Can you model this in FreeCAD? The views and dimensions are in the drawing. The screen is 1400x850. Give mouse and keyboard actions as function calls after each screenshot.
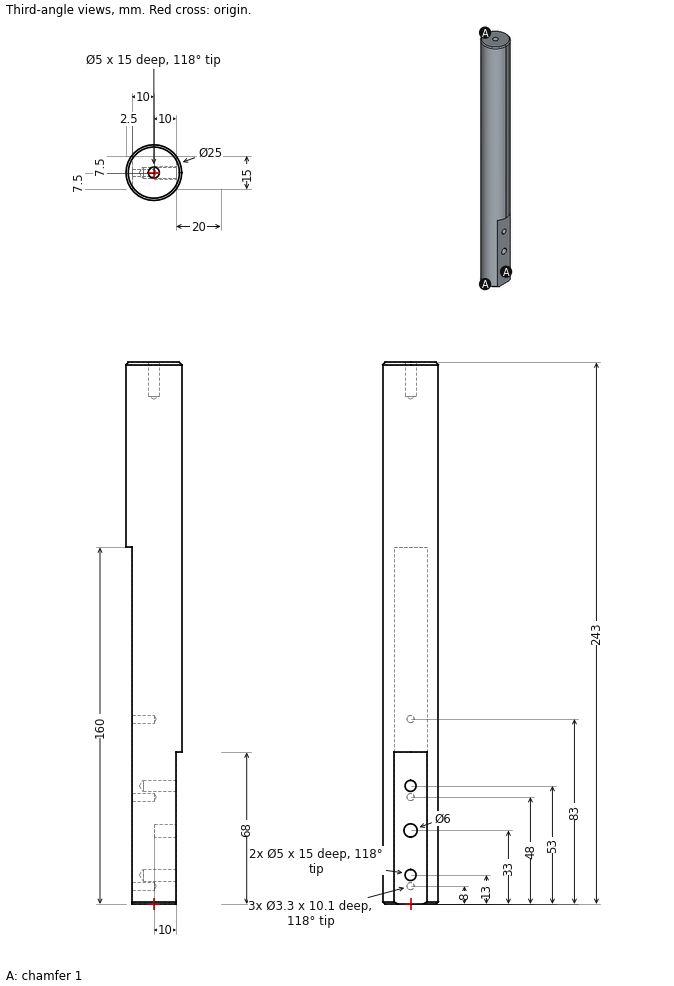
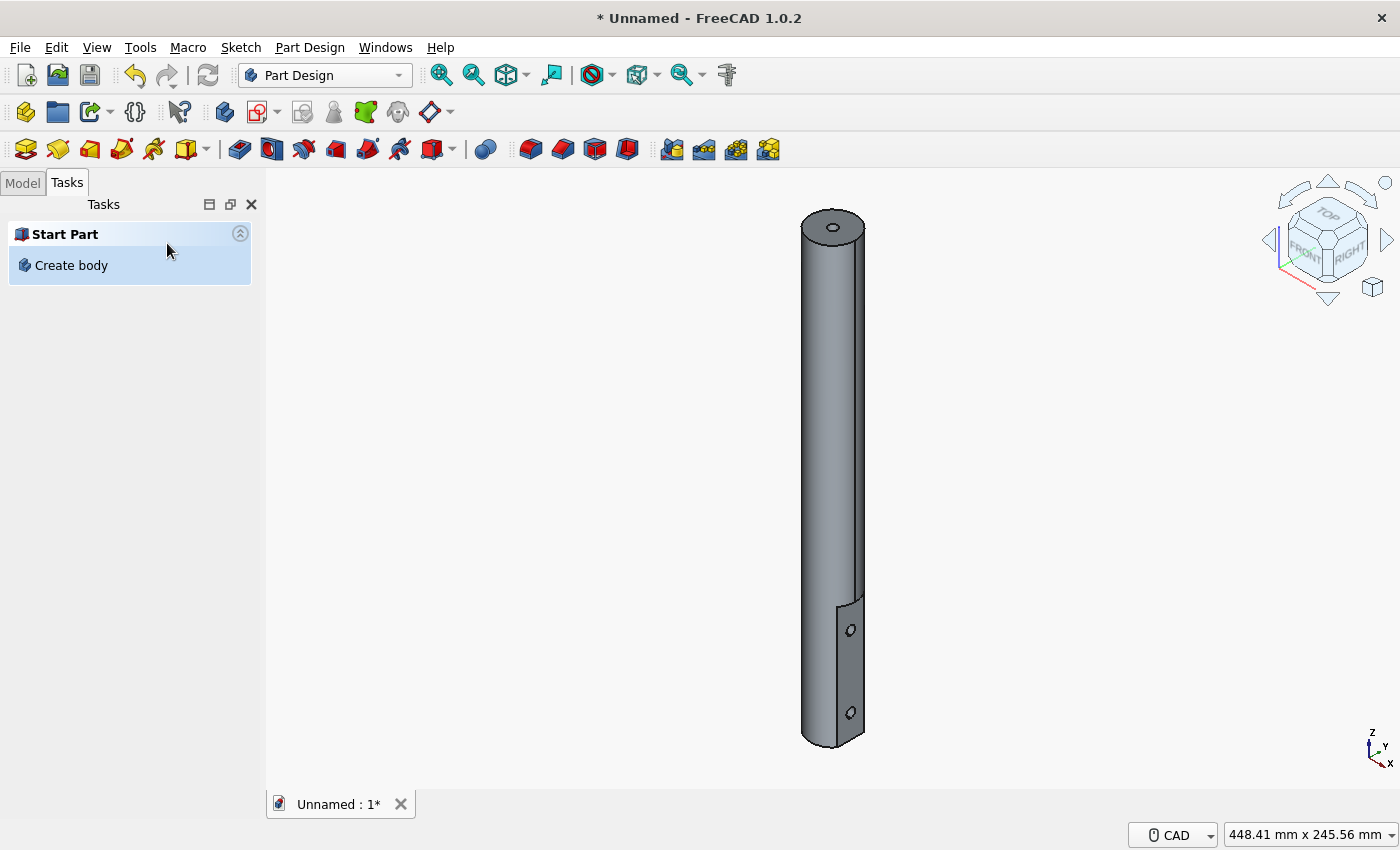
click(851, 668)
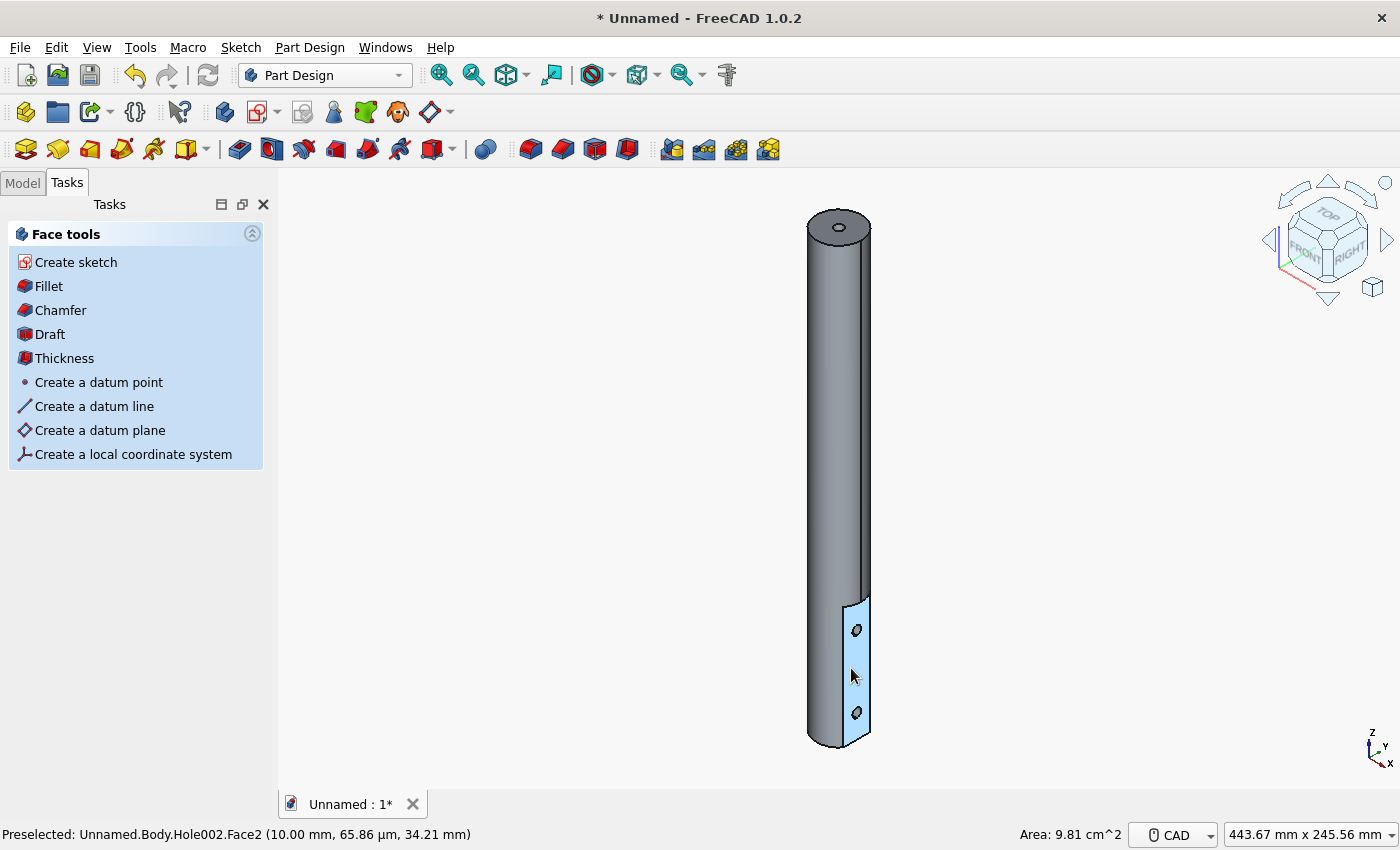
click(258, 112)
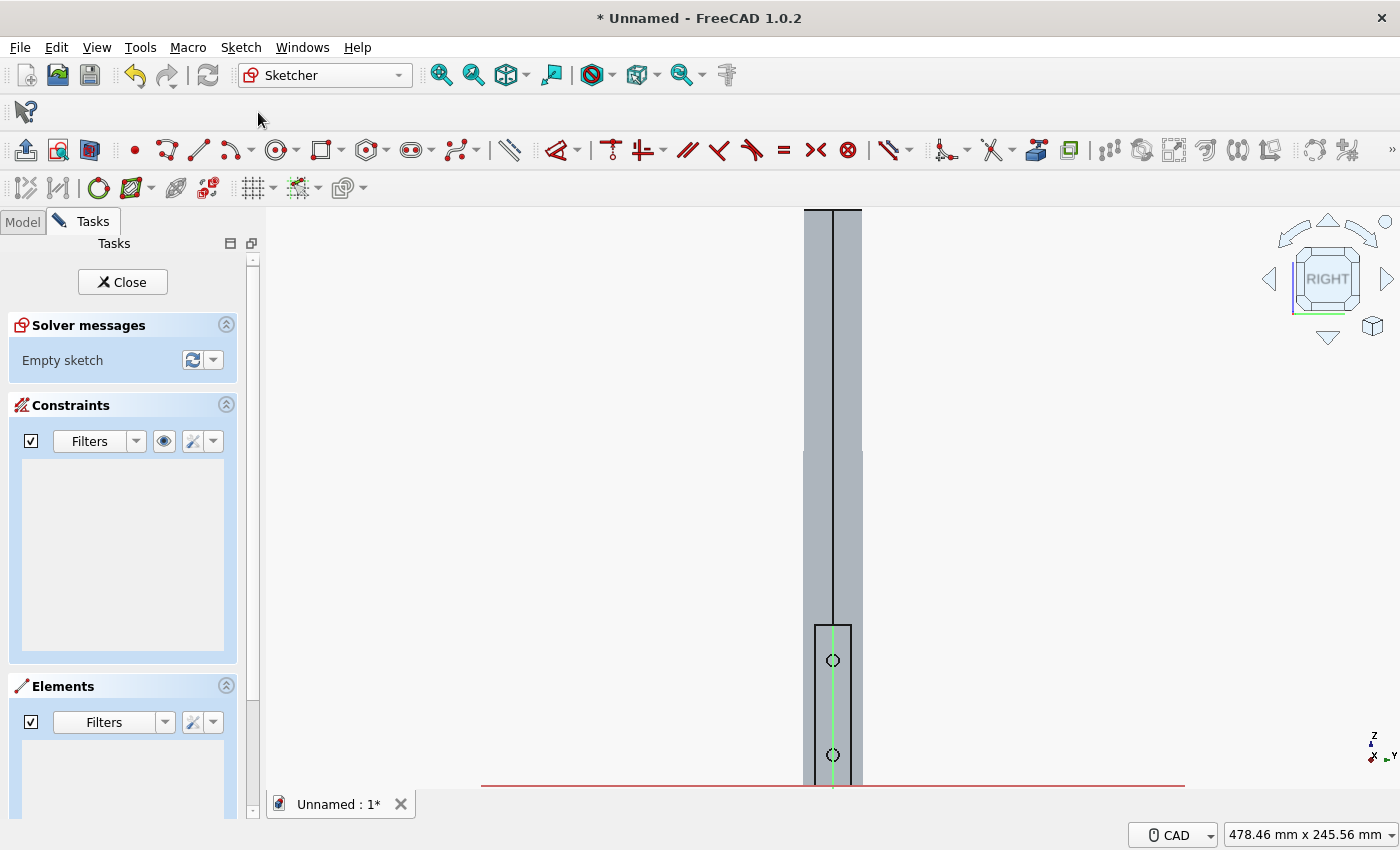
key(q)
key(s)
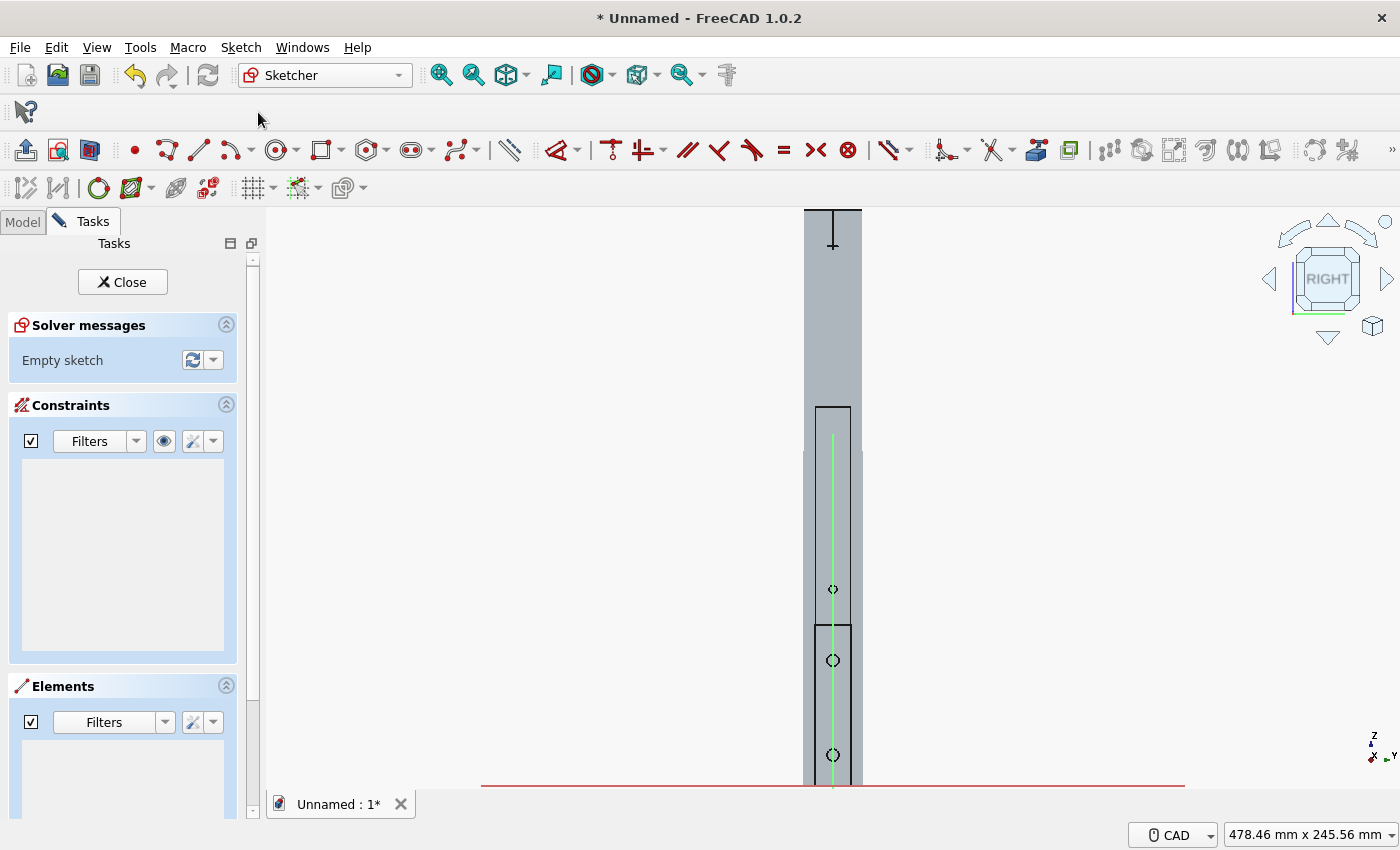
scroll(837, 719, up, 15)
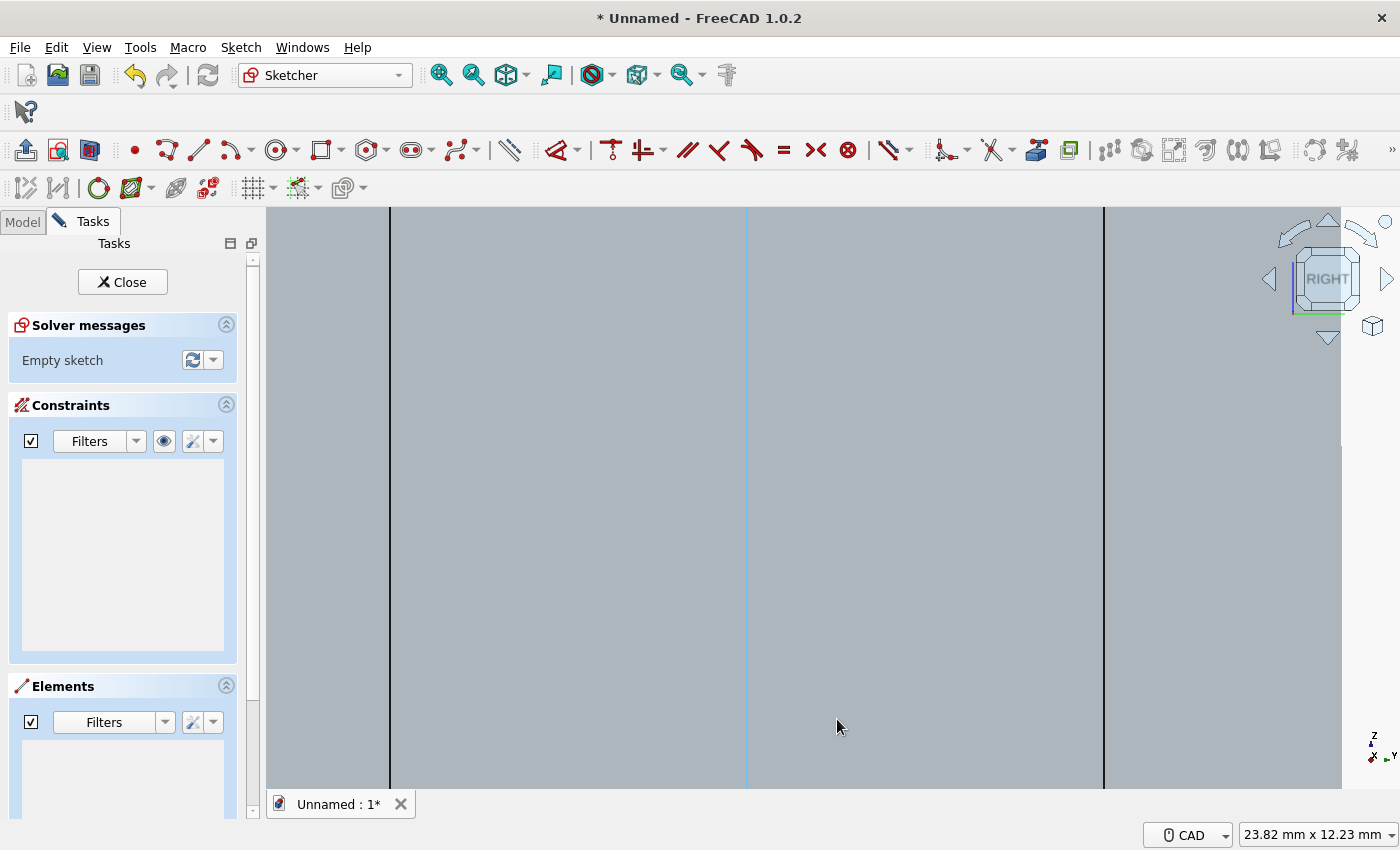
key(g)
key(c)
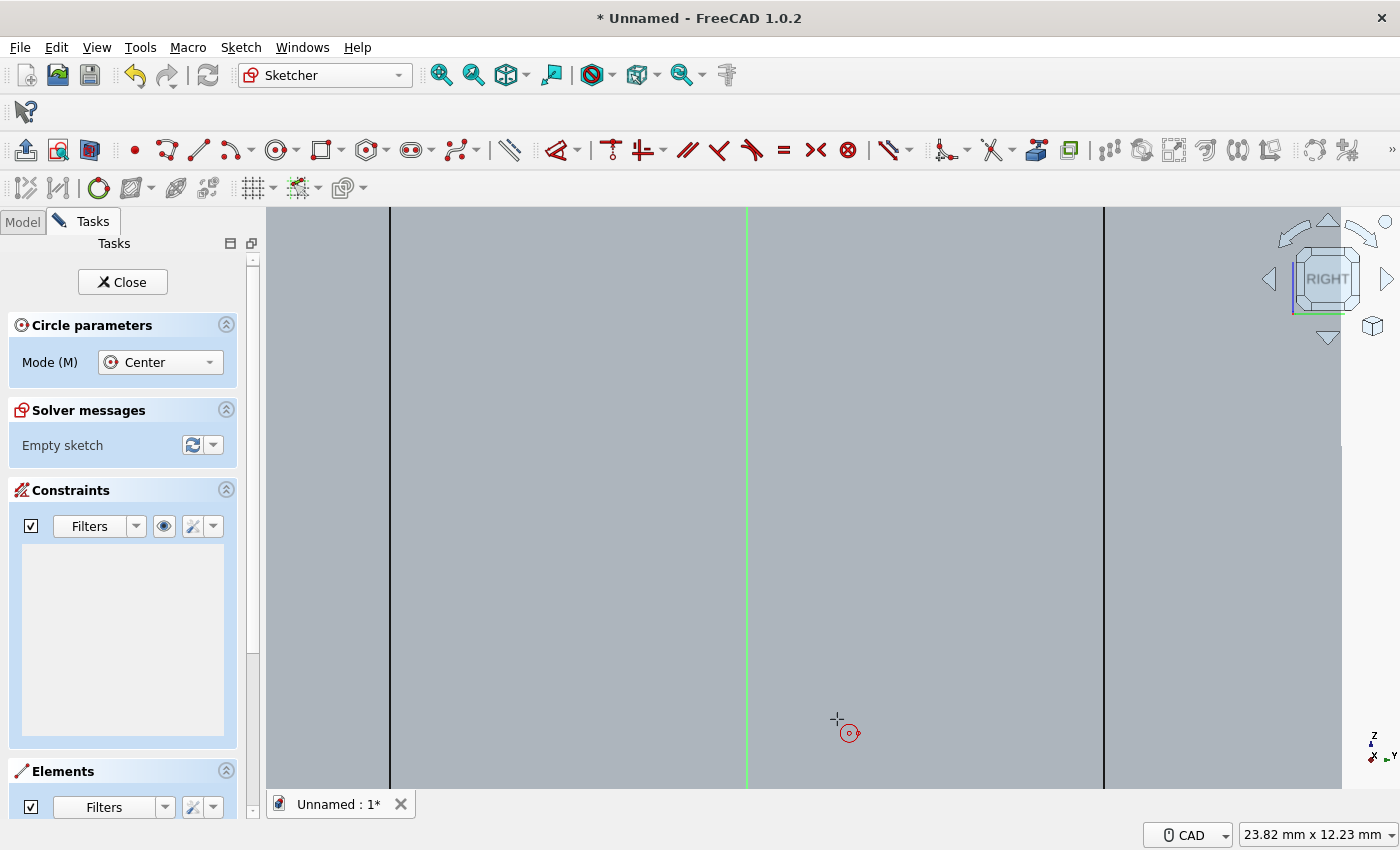
click(747, 476)
click(848, 375)
key(Escape)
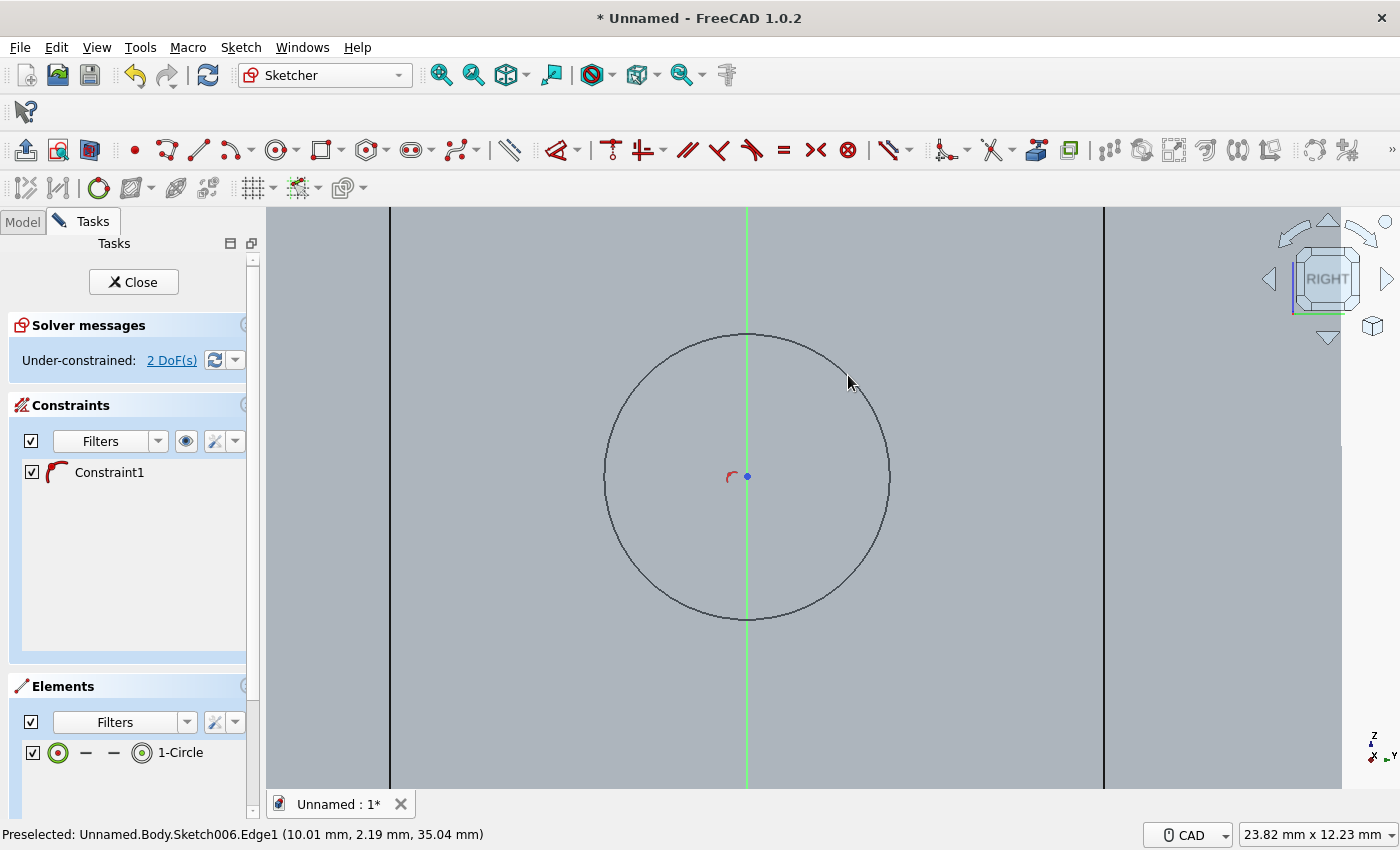
key(d)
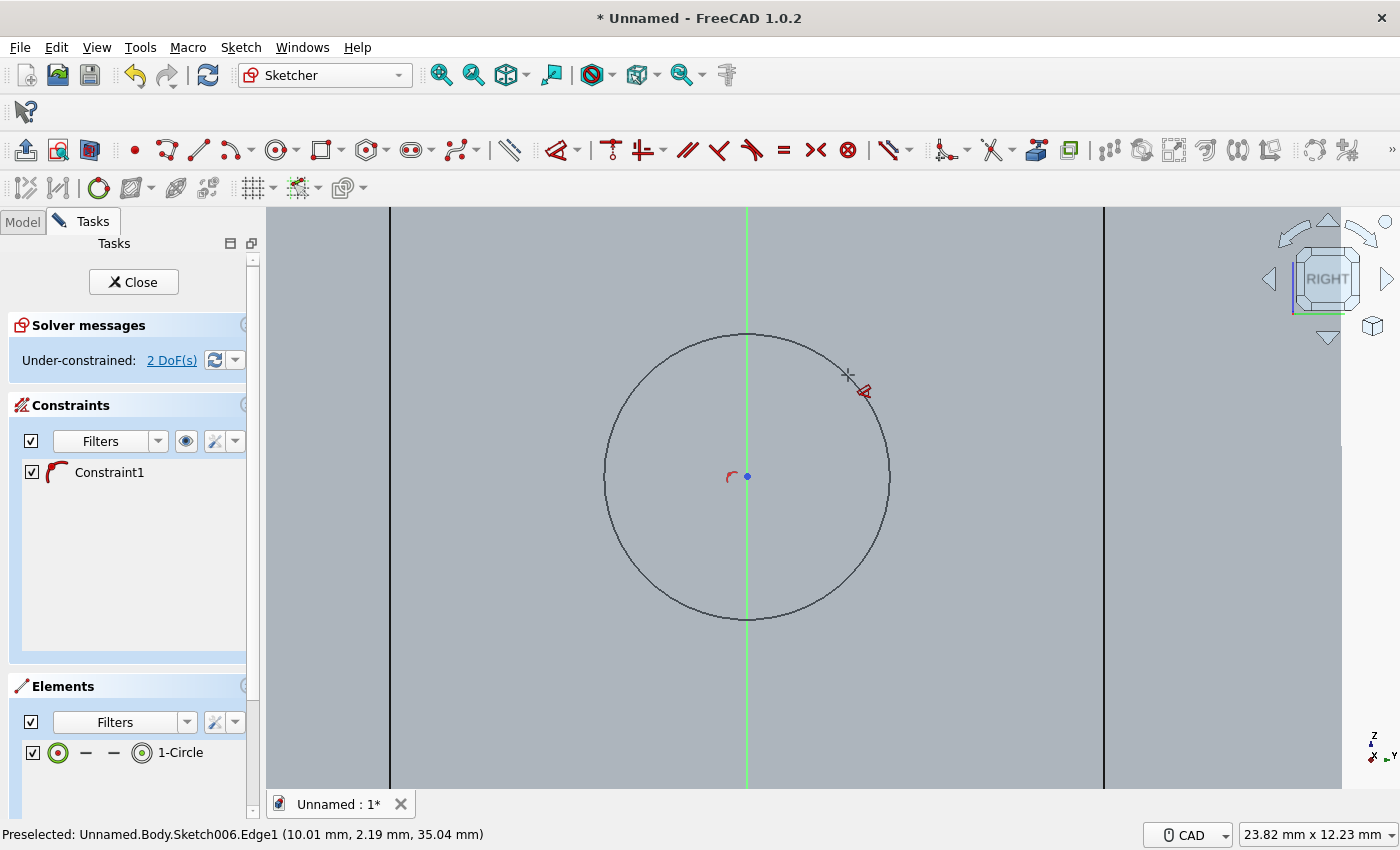
click(848, 376)
click(871, 353)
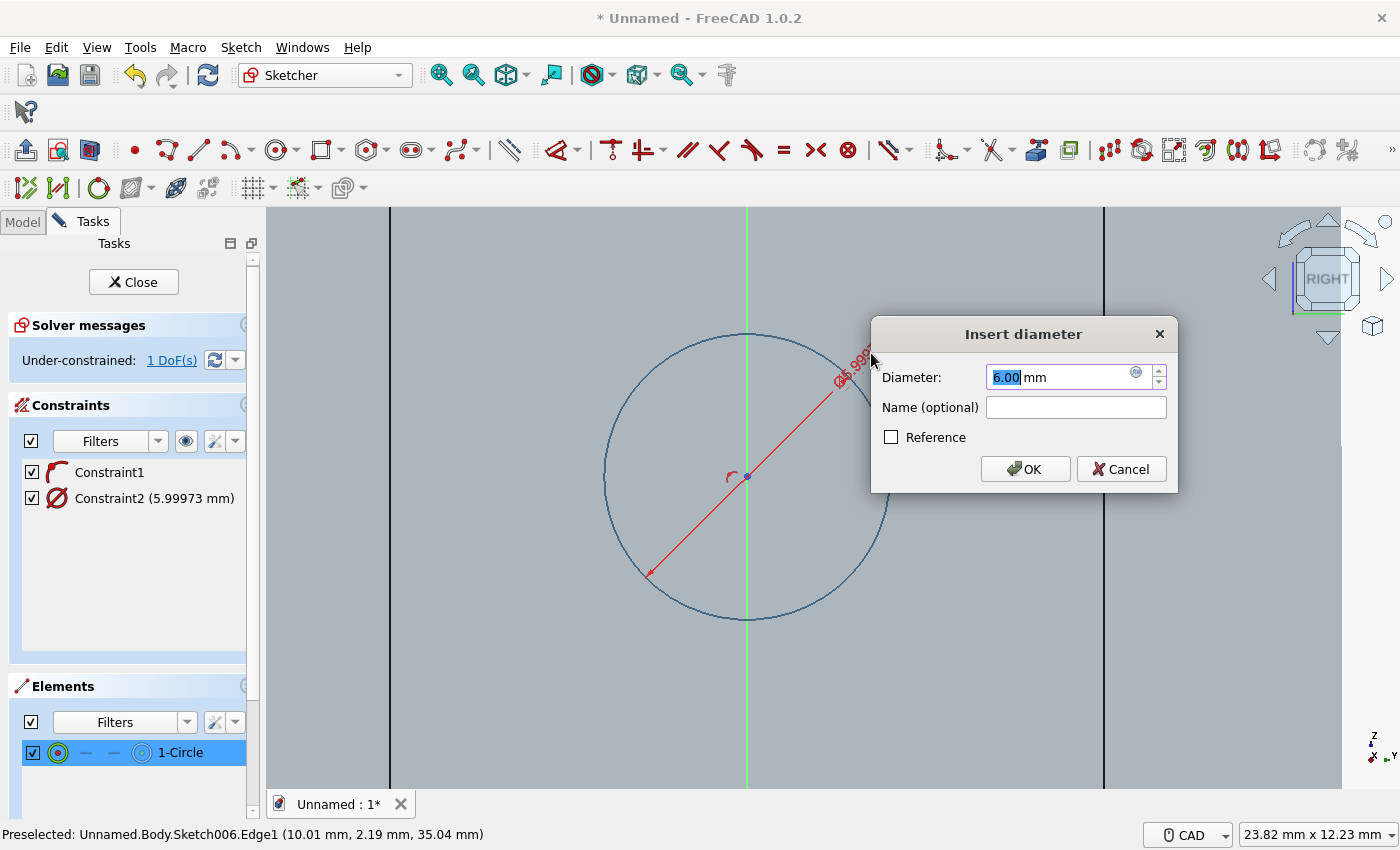
text(6)
key(Return)